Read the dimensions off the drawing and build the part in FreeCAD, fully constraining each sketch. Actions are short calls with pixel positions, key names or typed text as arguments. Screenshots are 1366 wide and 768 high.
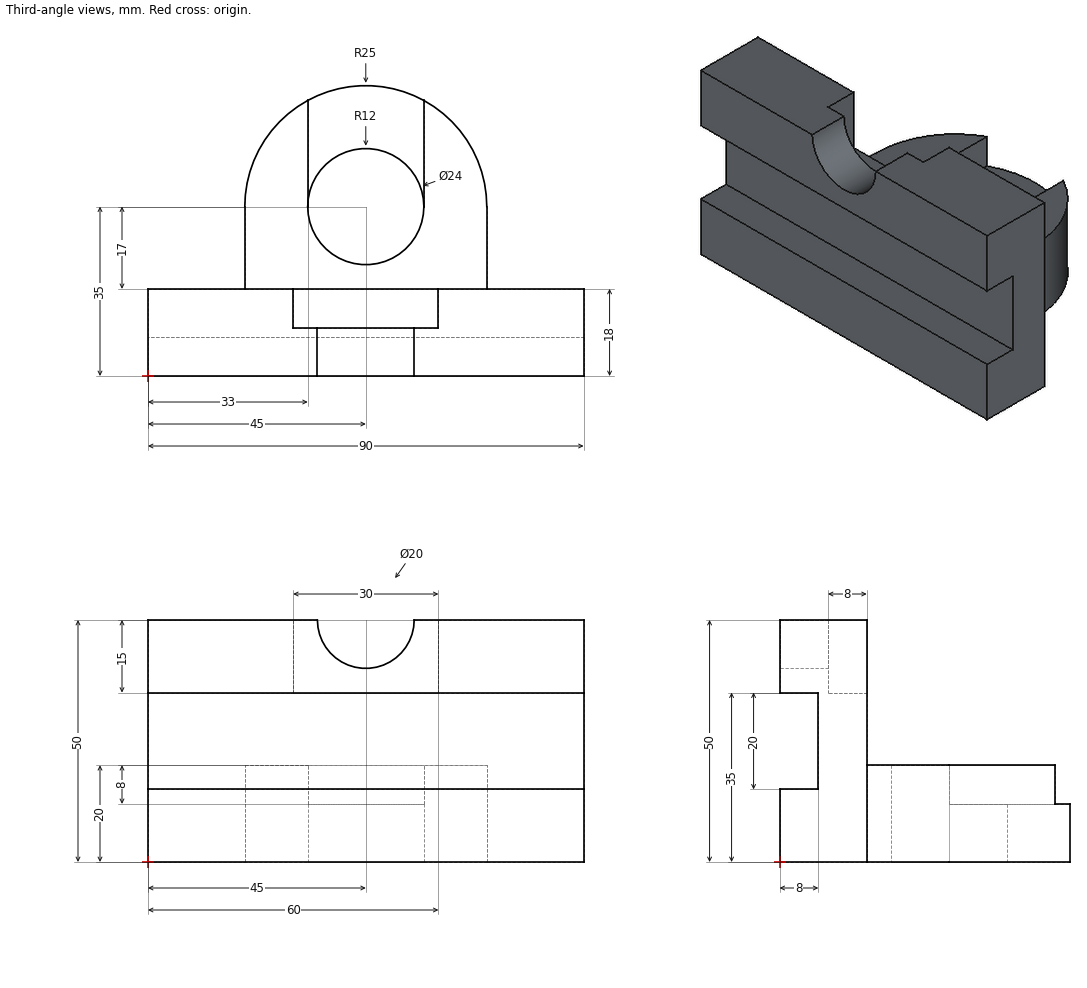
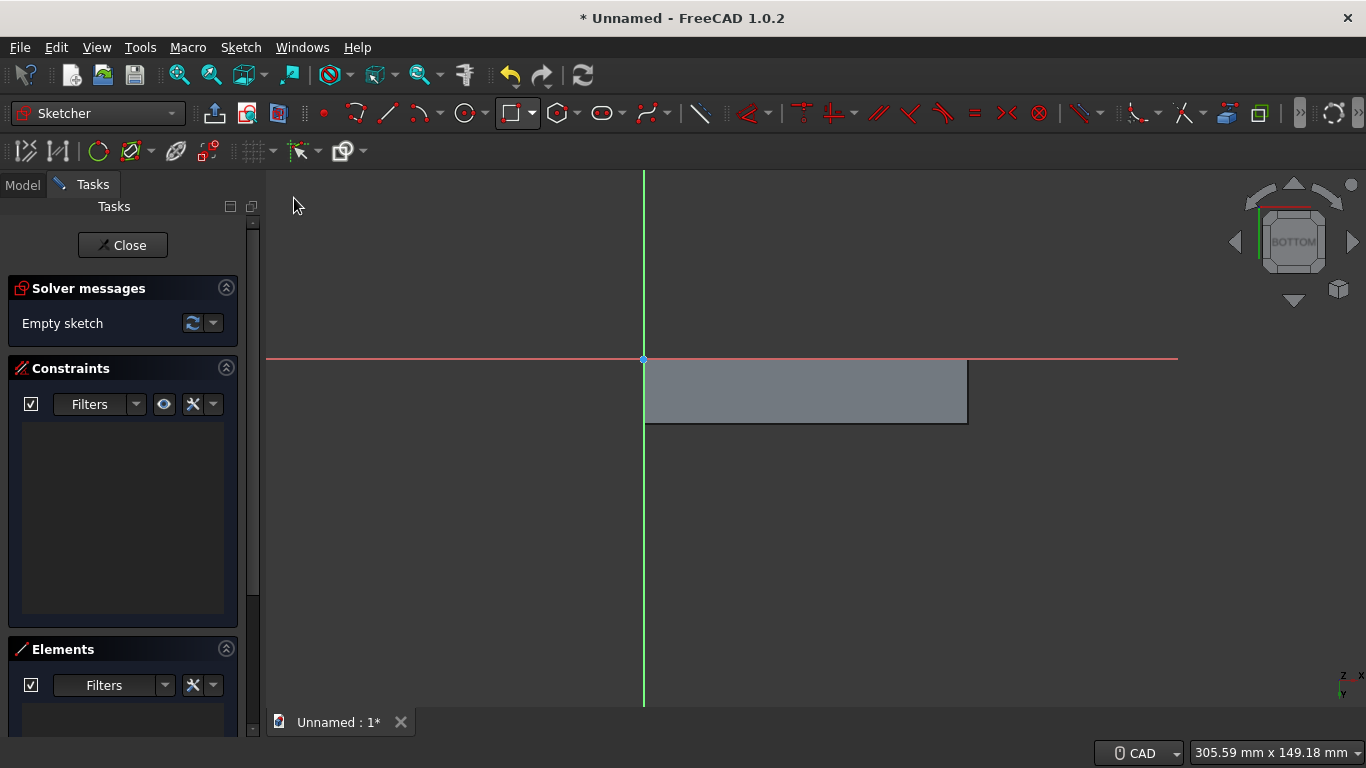
scroll(815, 526, up, 2)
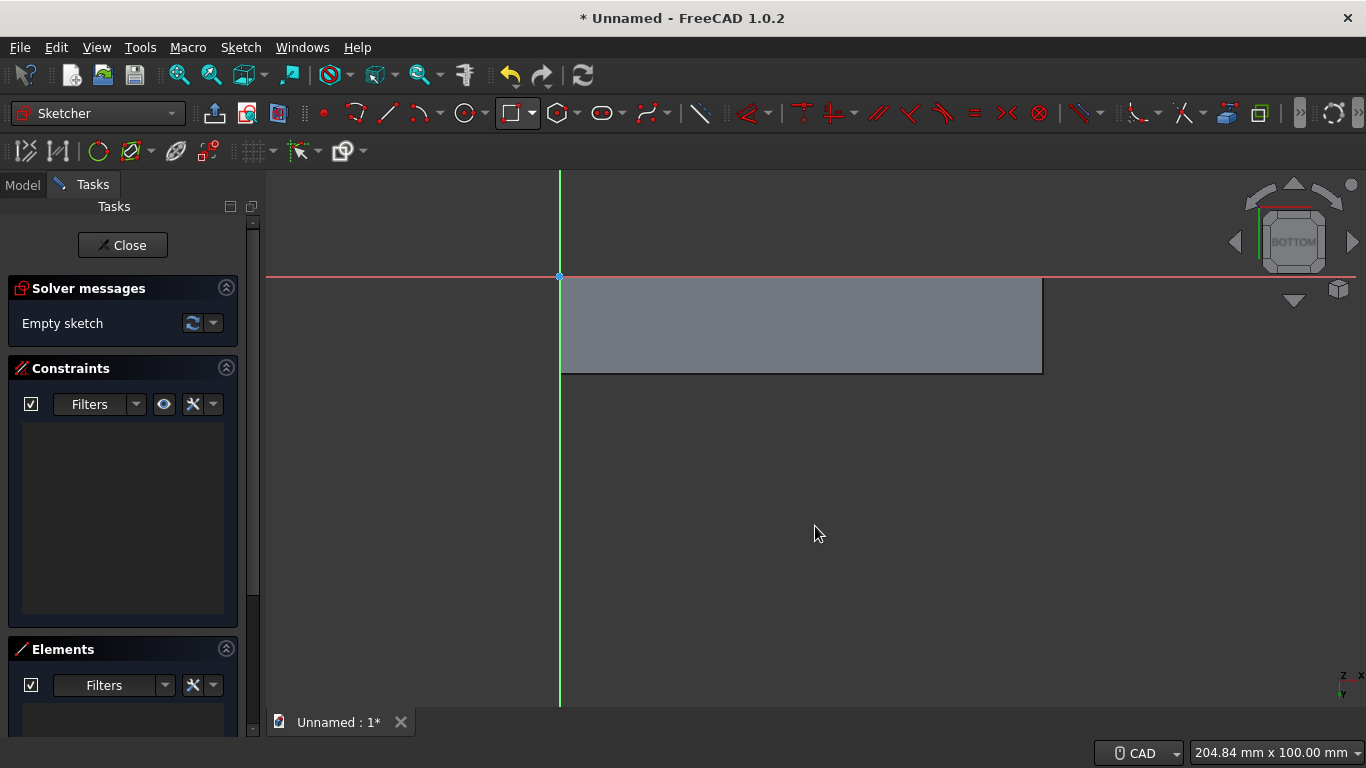
key(g)
key(m)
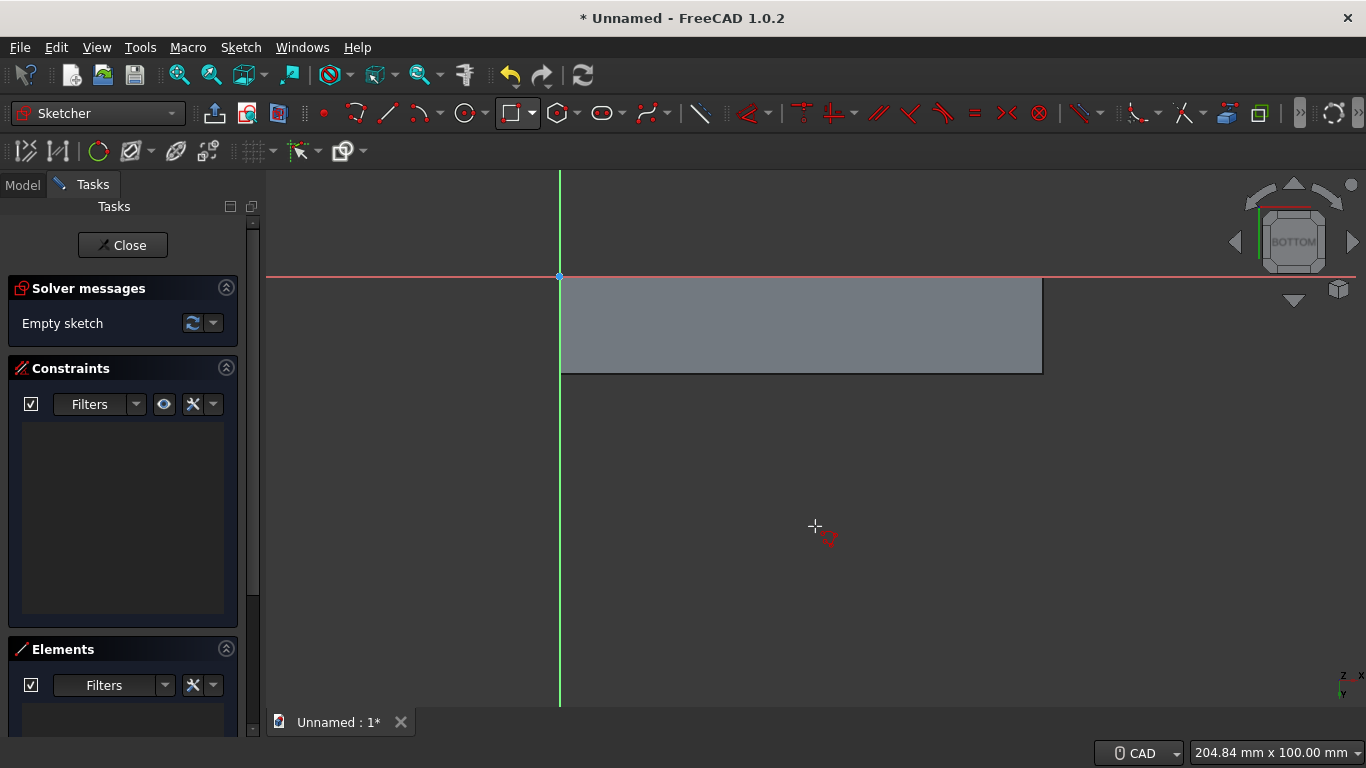
click(667, 465)
click(667, 374)
click(935, 374)
click(935, 465)
right_click(935, 465)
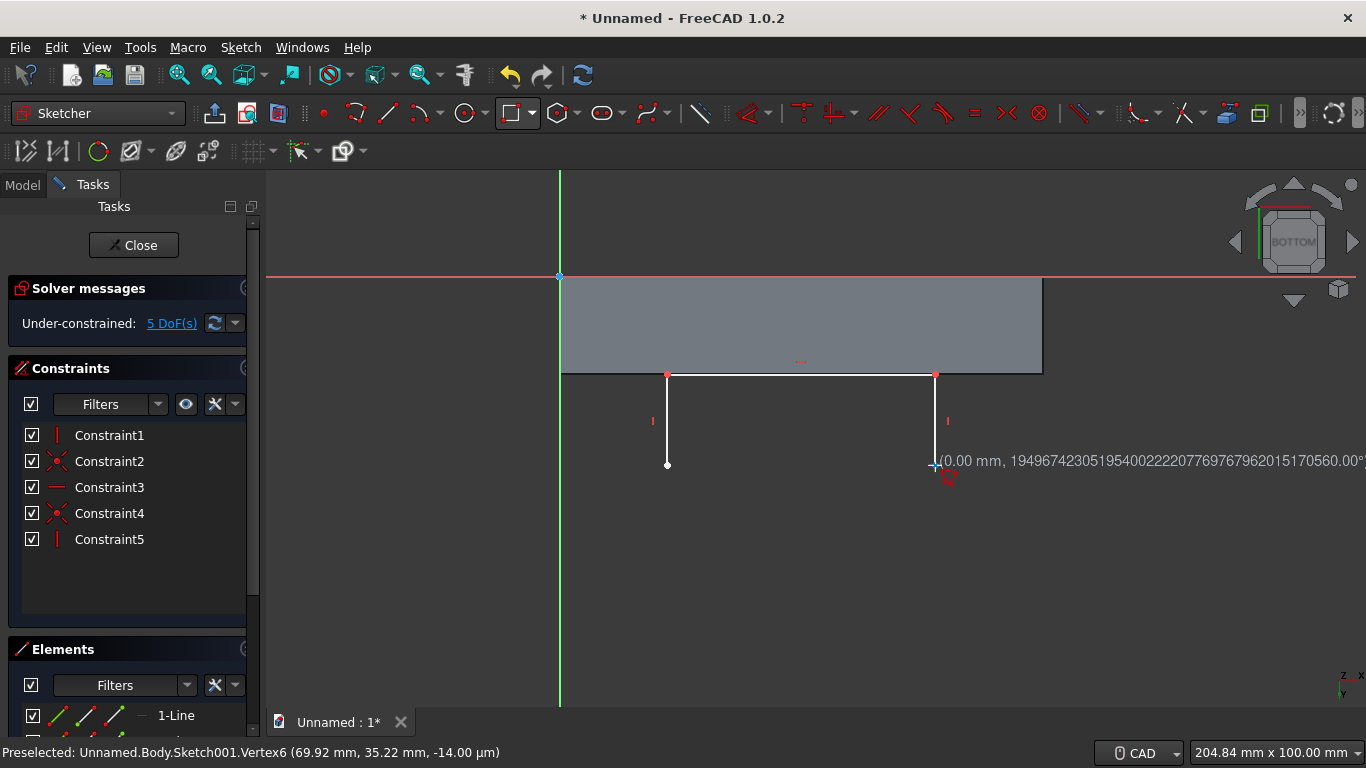
key(g)
key(3)
key(a)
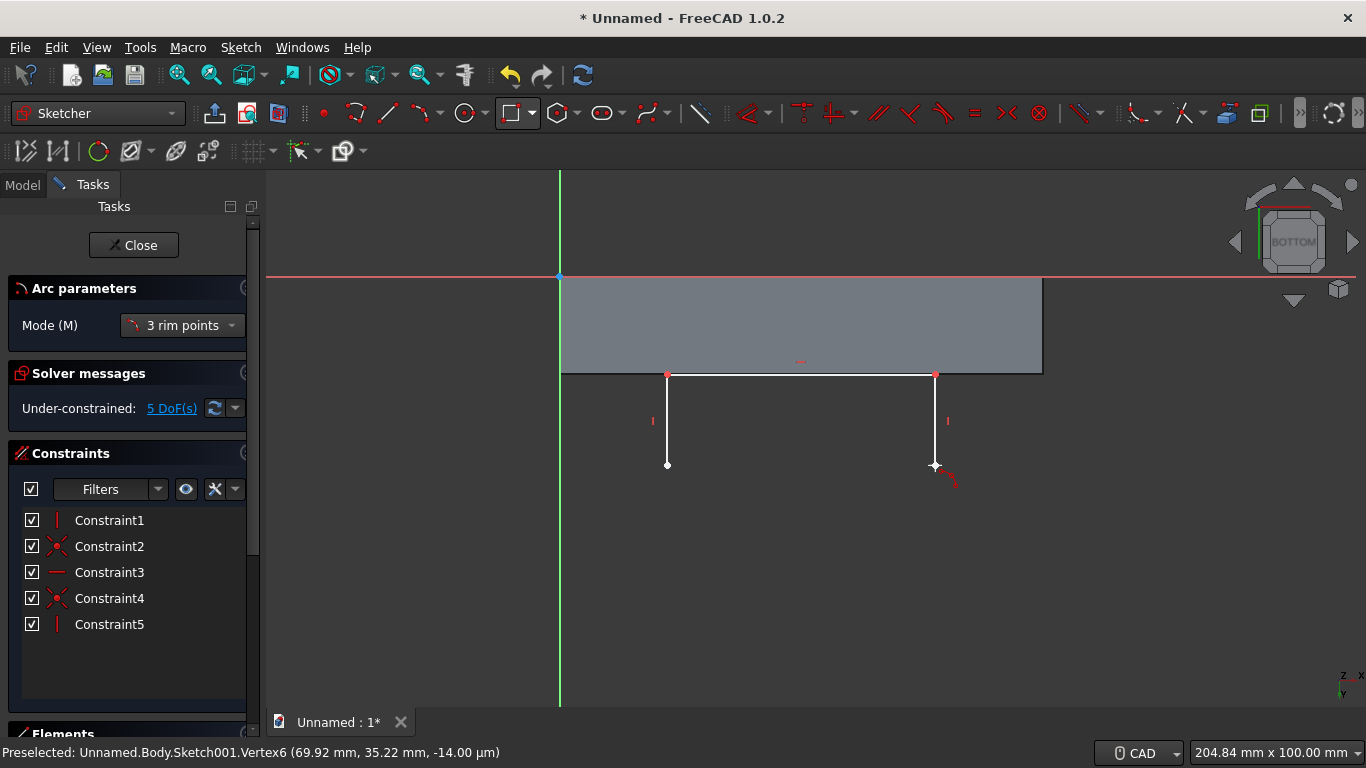
click(935, 466)
click(667, 466)
click(801, 599)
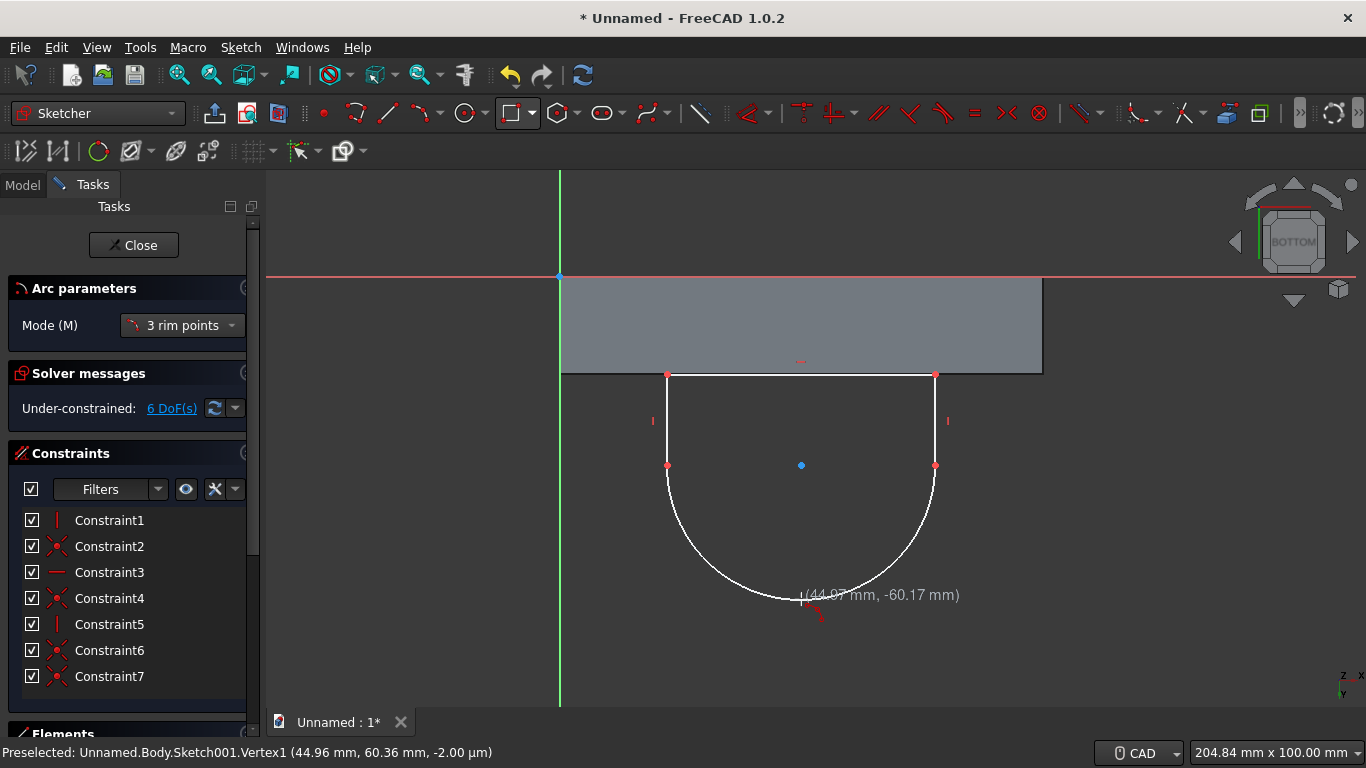
click(466, 114)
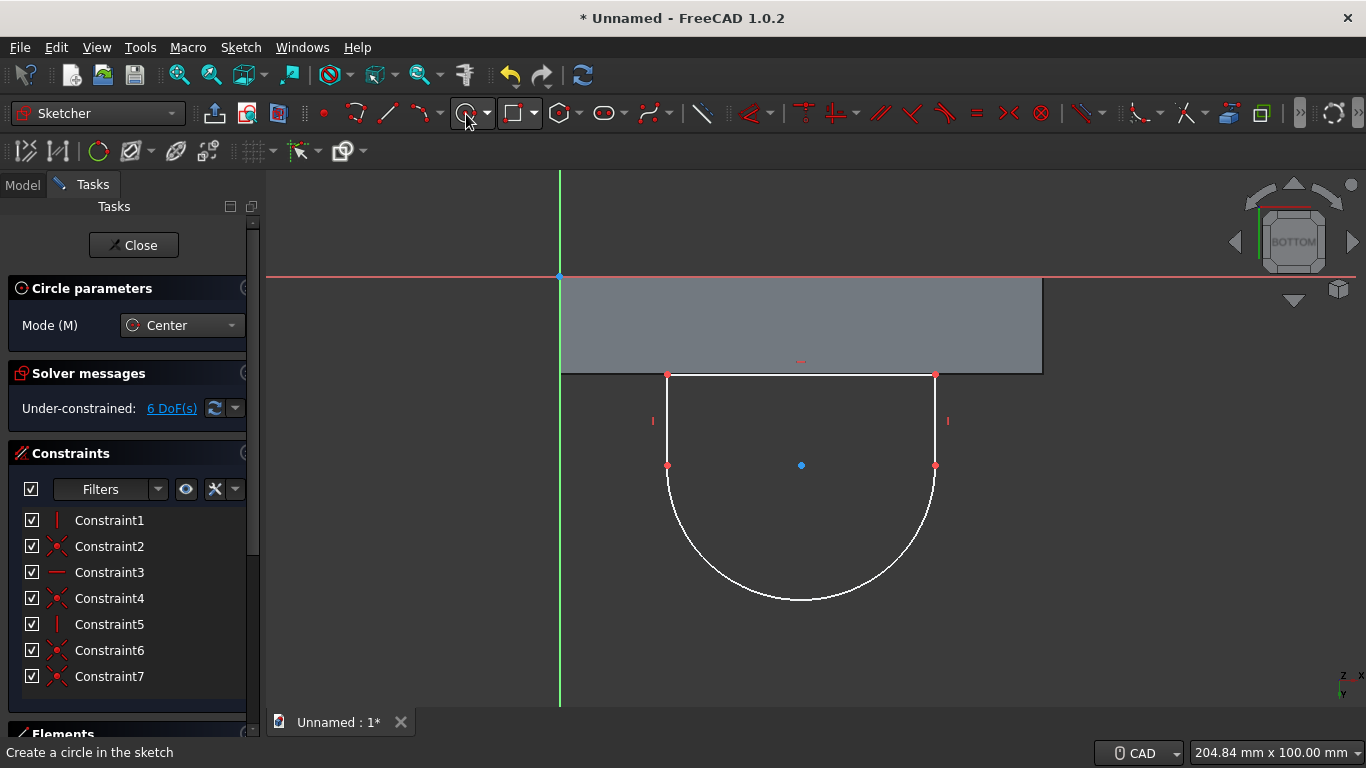
click(801, 465)
move(847, 419)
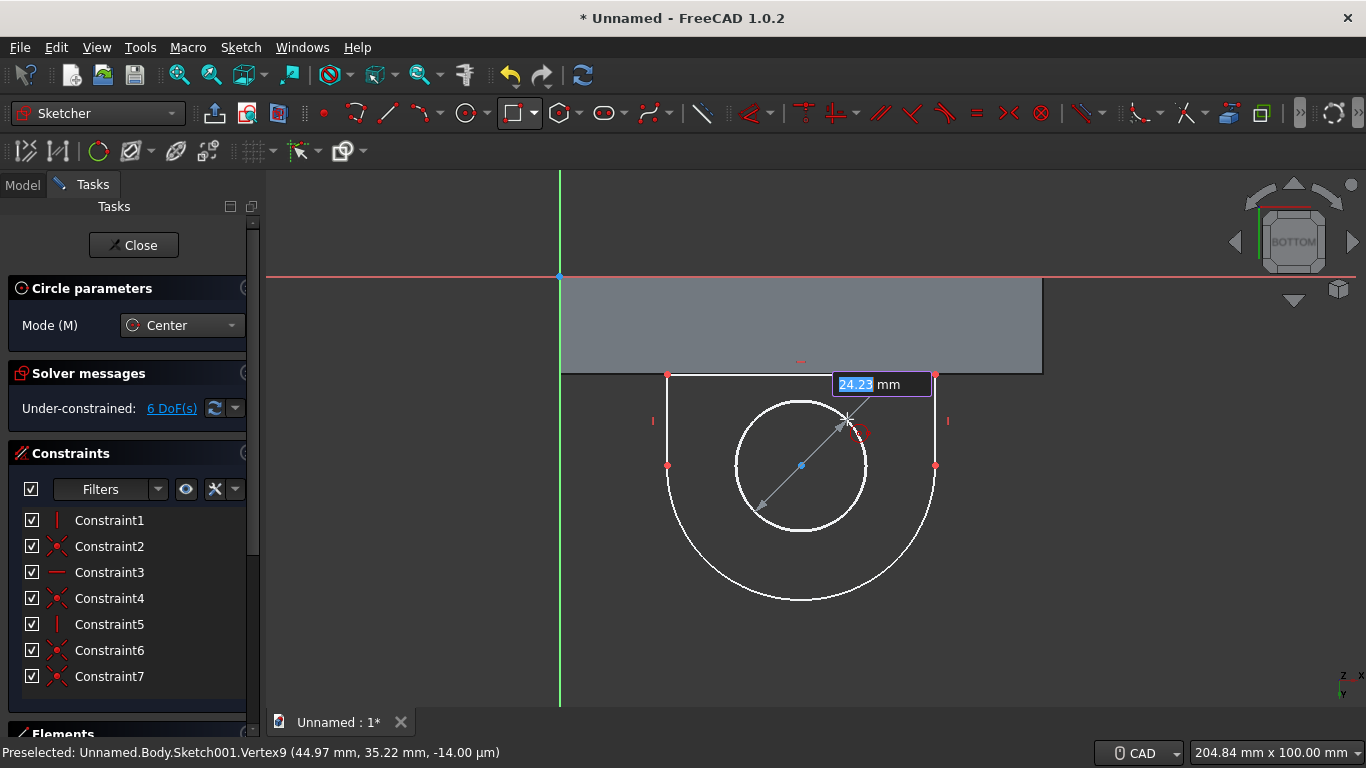
text(24)
key(Return)
key(Escape)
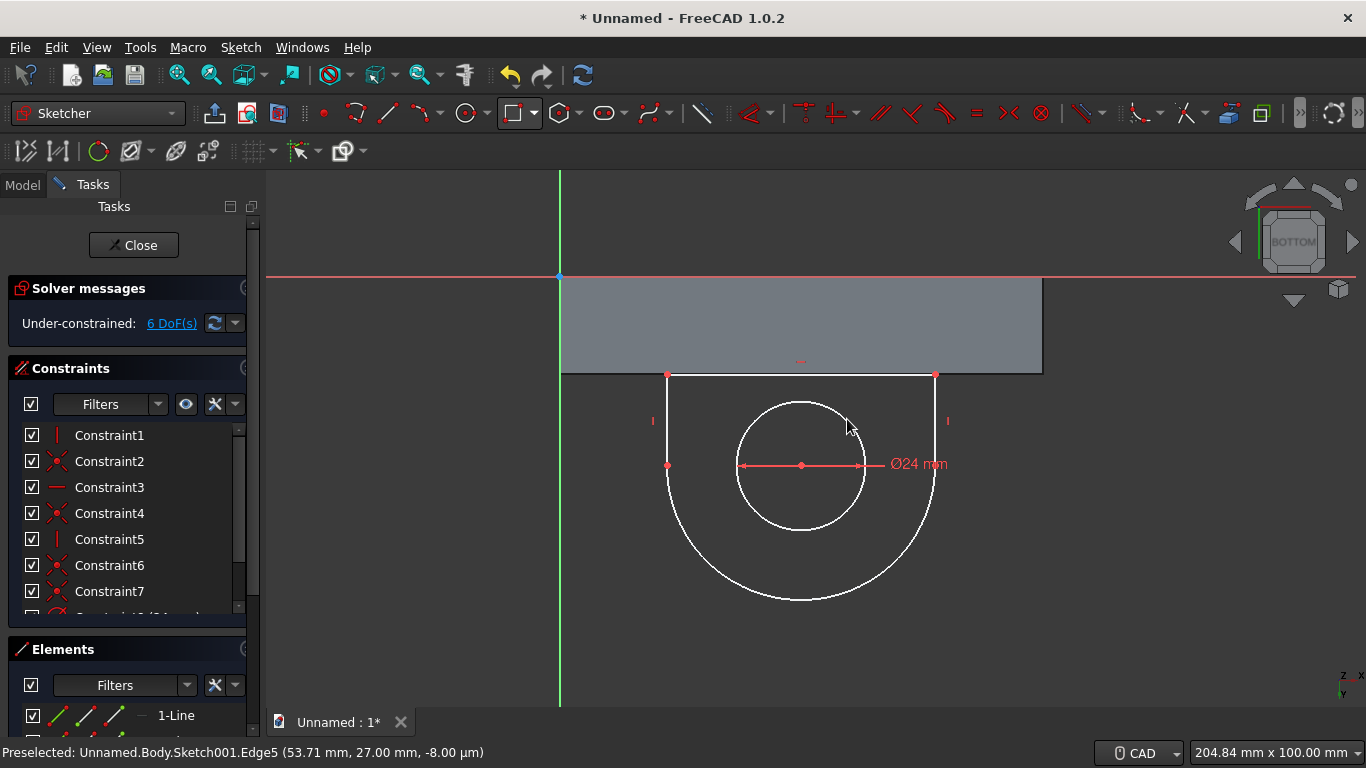
click(667, 439)